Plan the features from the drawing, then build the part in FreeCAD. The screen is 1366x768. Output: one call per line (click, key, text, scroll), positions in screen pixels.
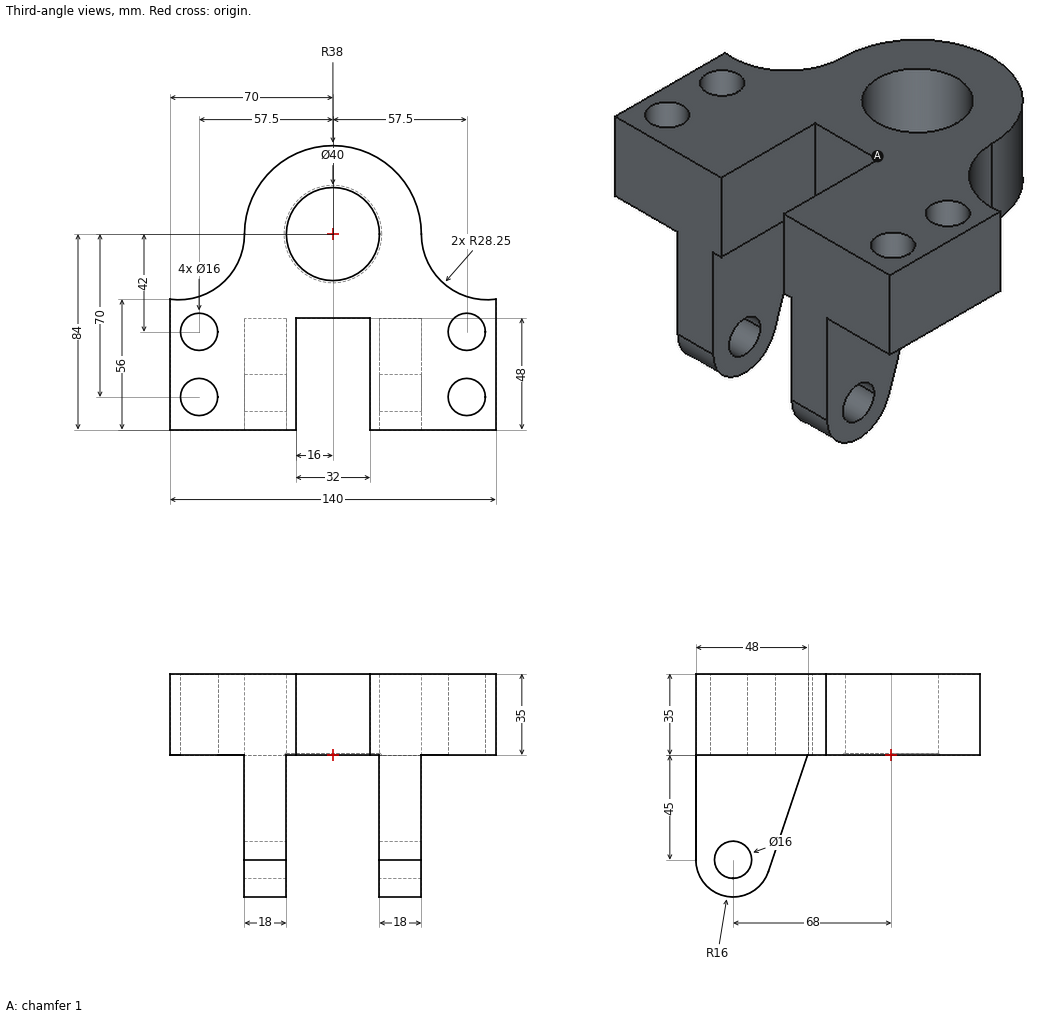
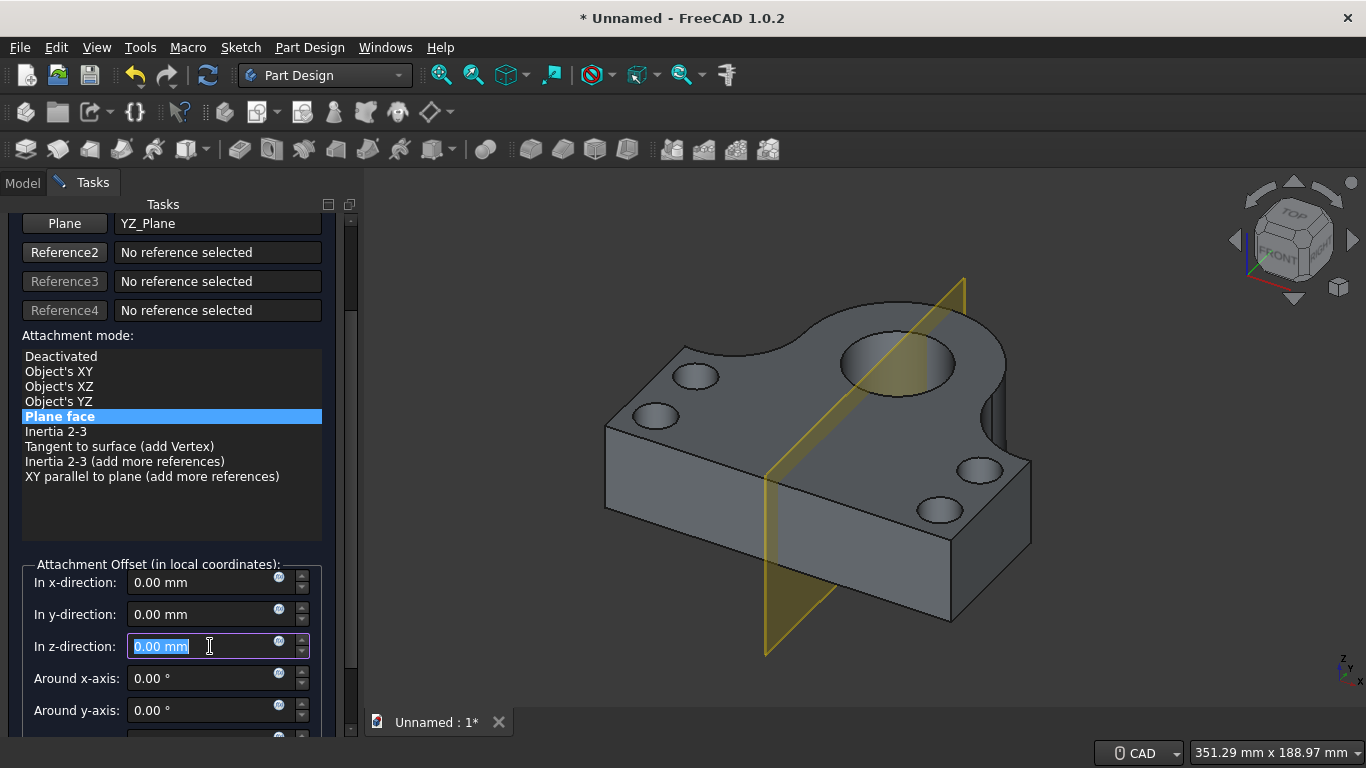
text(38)
key(Tab)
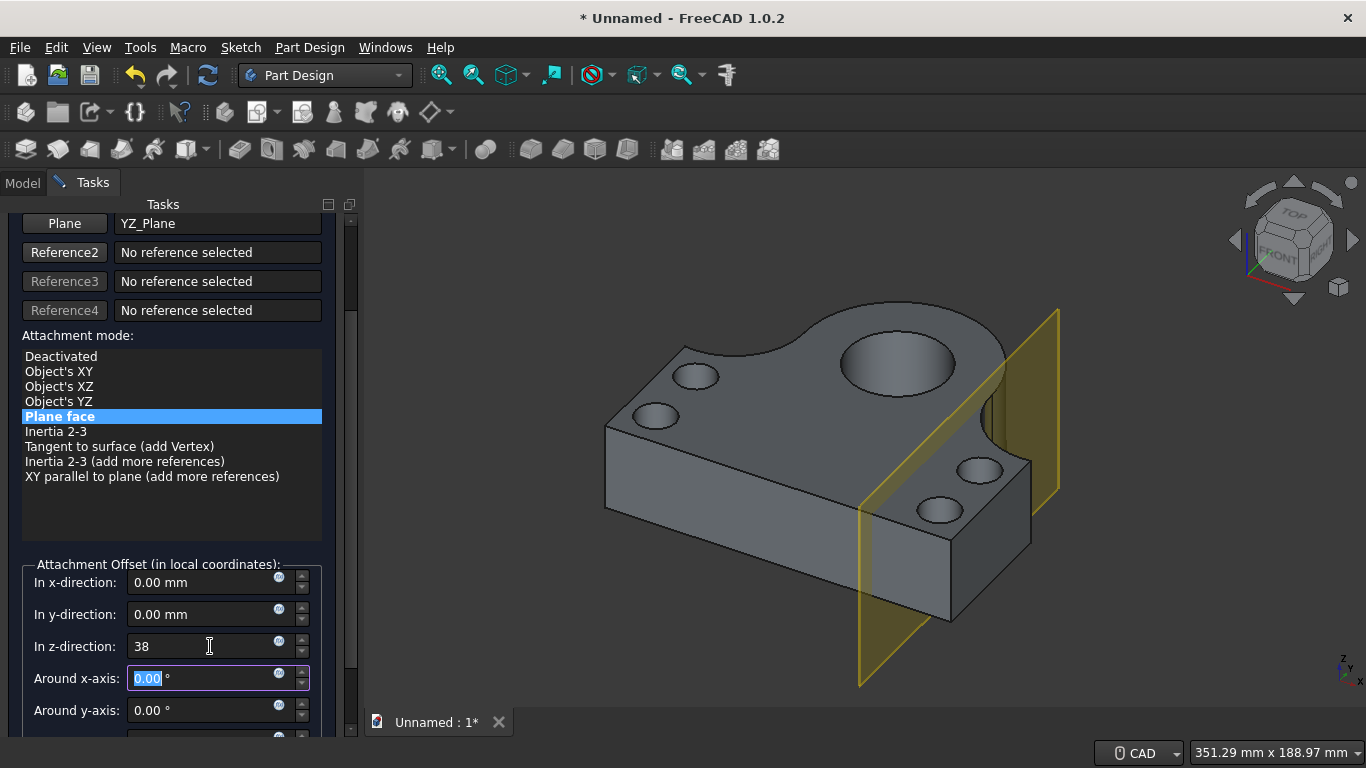
scroll(351, 475, up, 3)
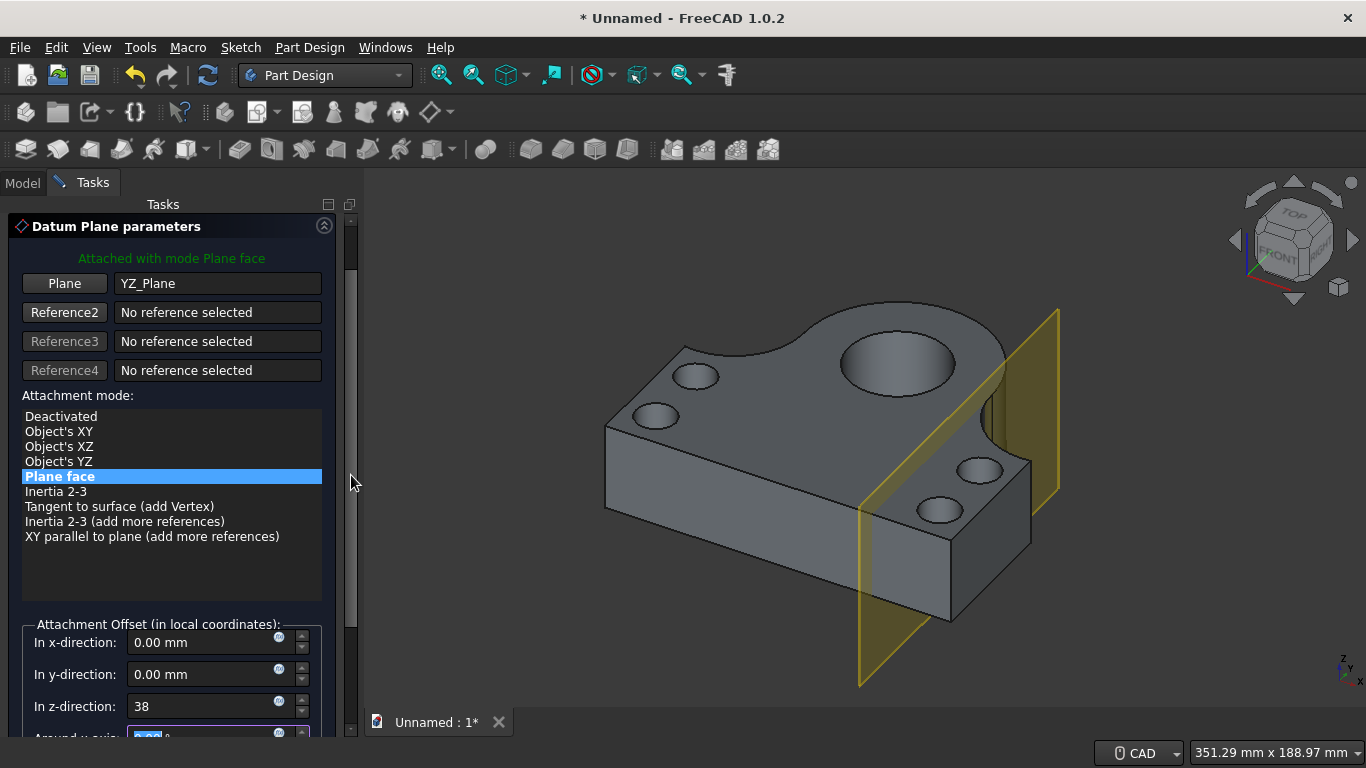
click(124, 243)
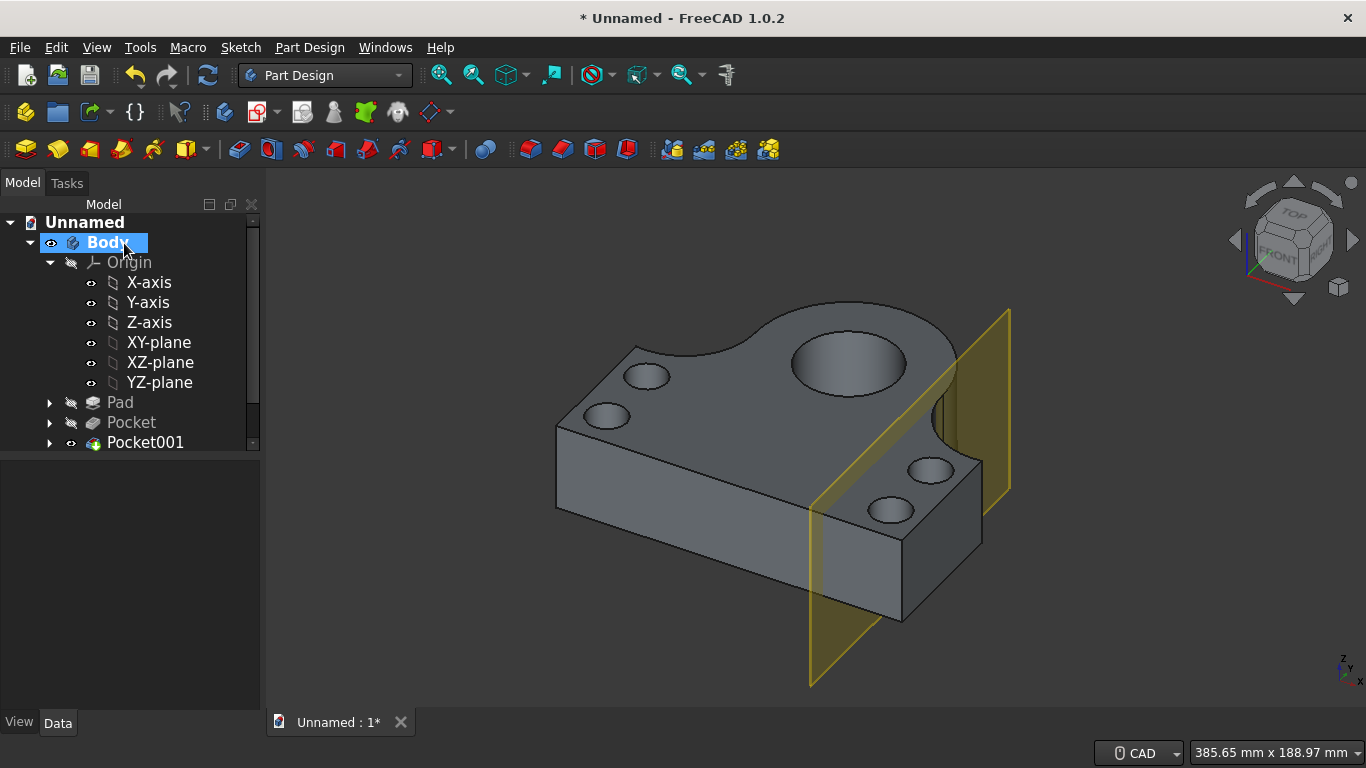
scroll(100, 338, down, 3)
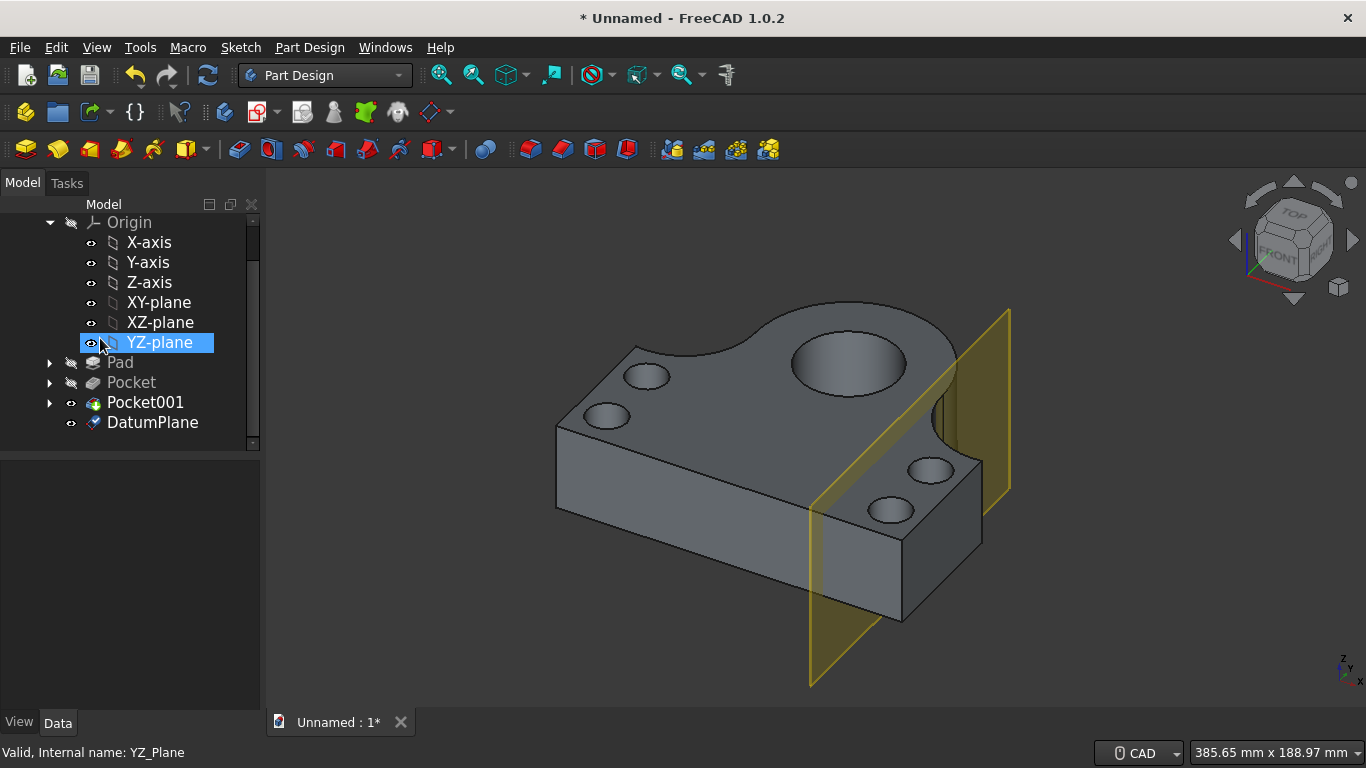
click(116, 423)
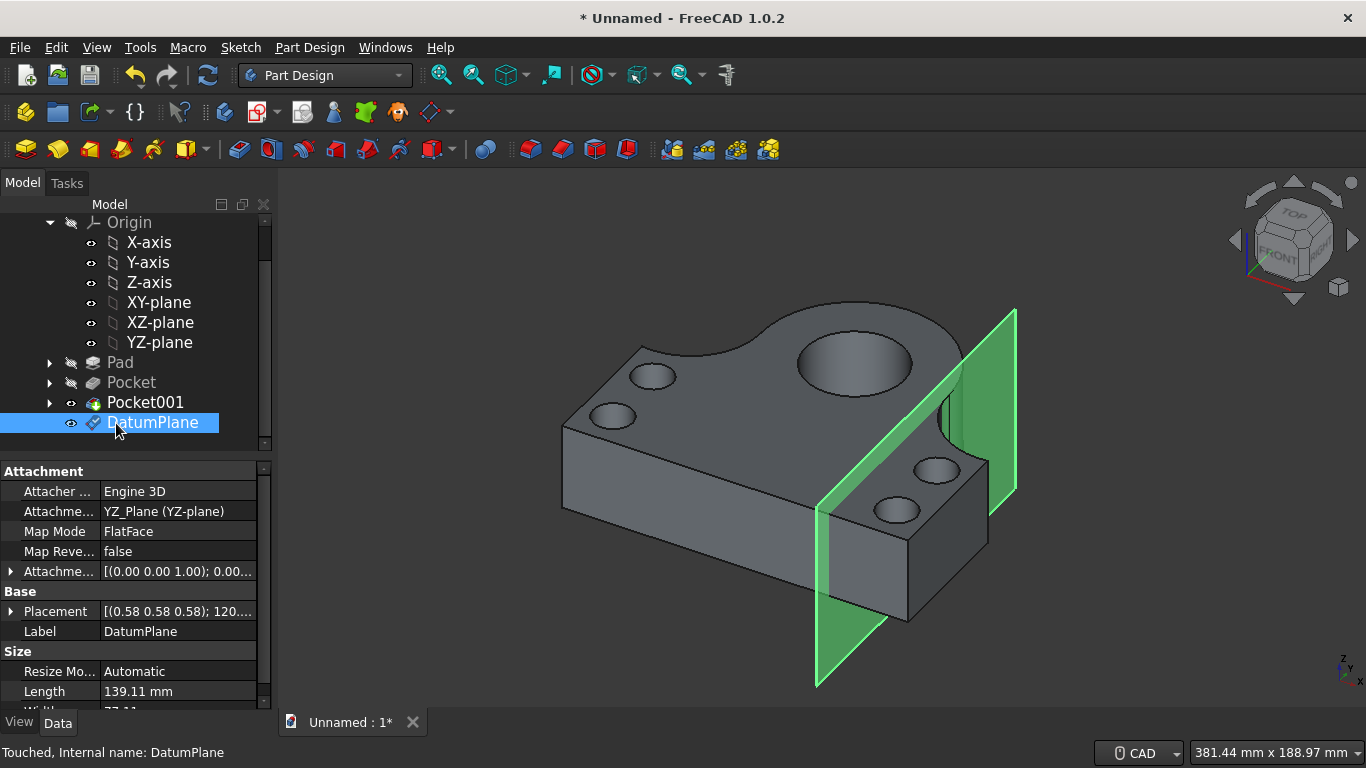
click(258, 112)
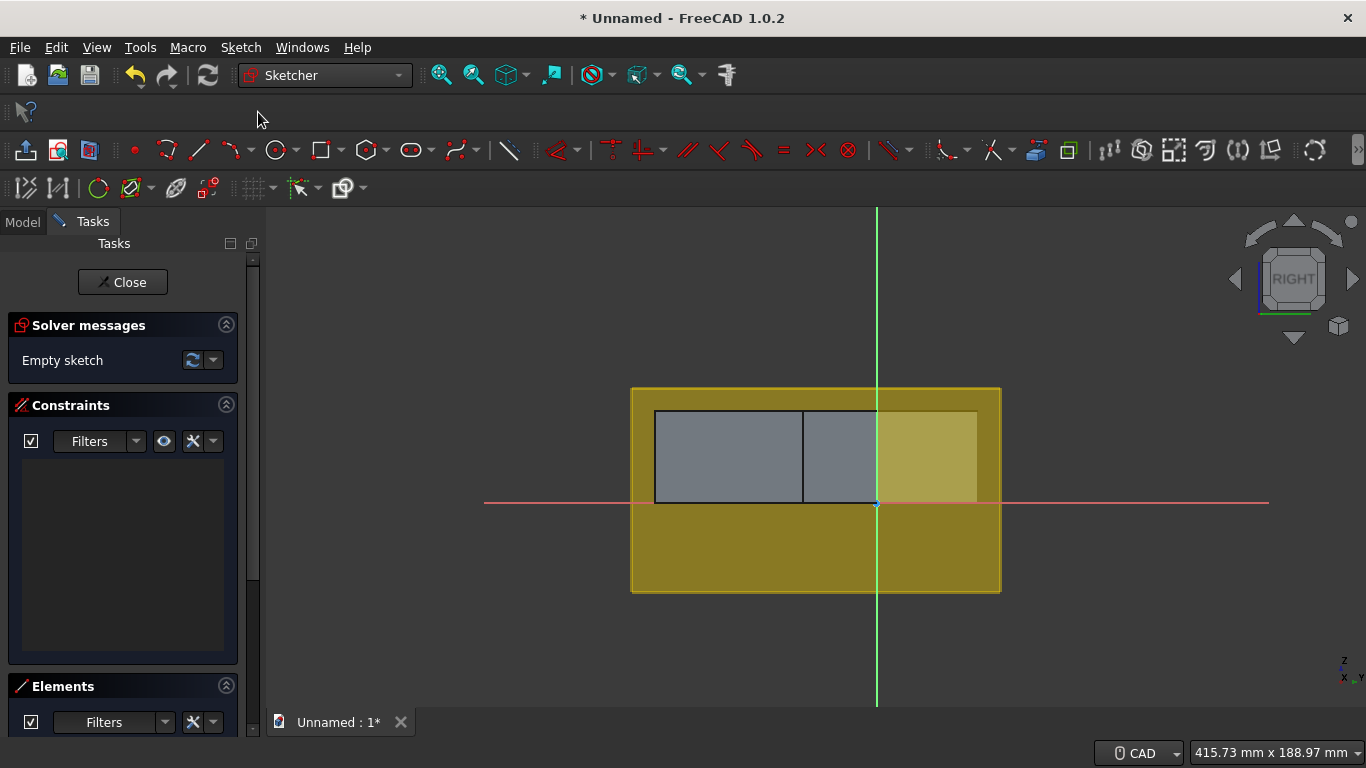
key(q)
key(s)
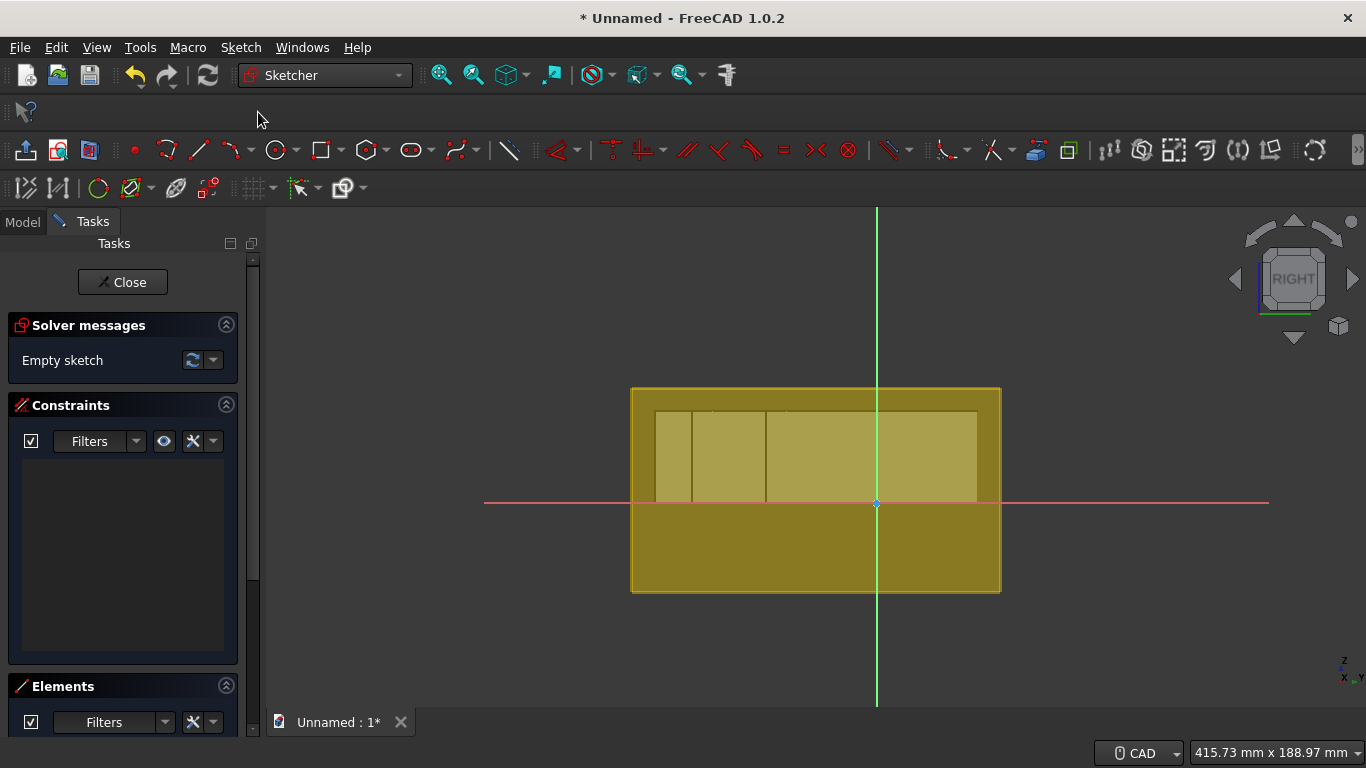
scroll(788, 679, up, 3)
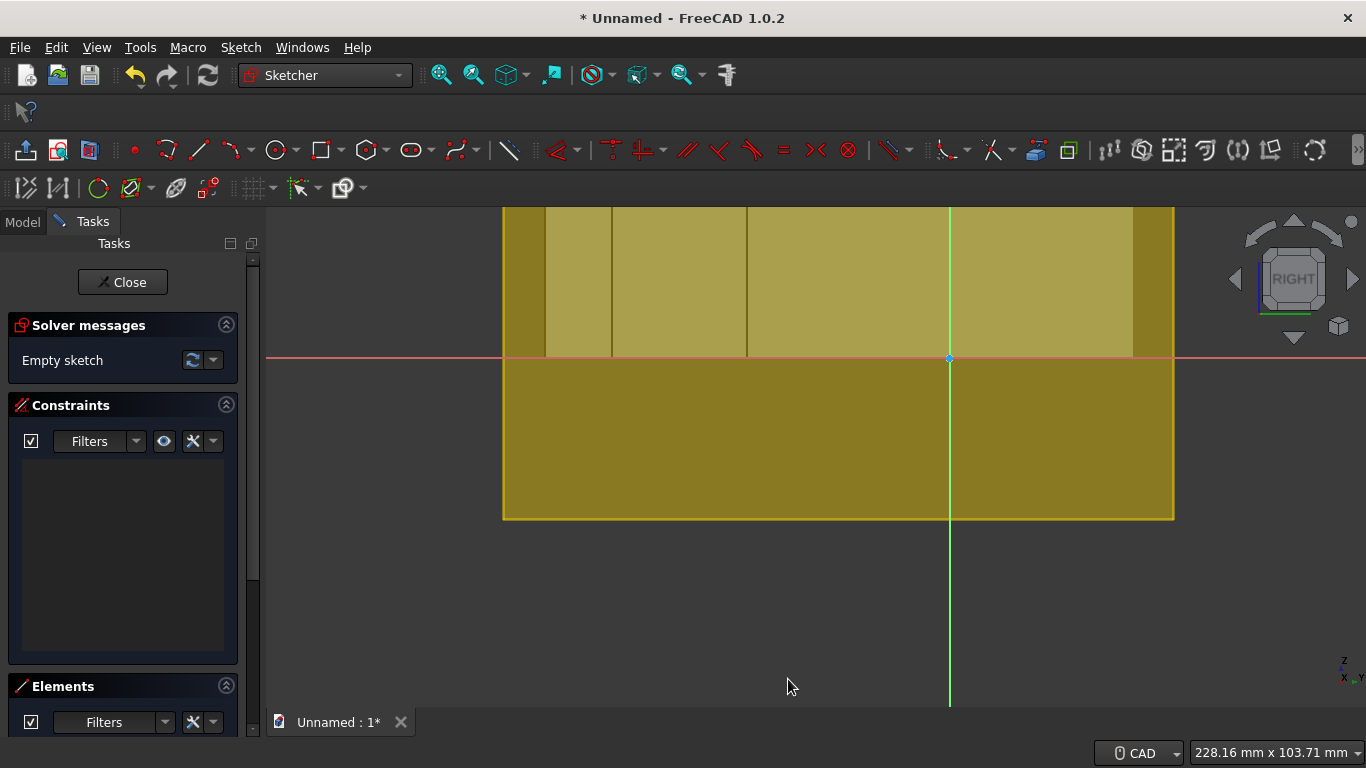
key(g)
key(m)